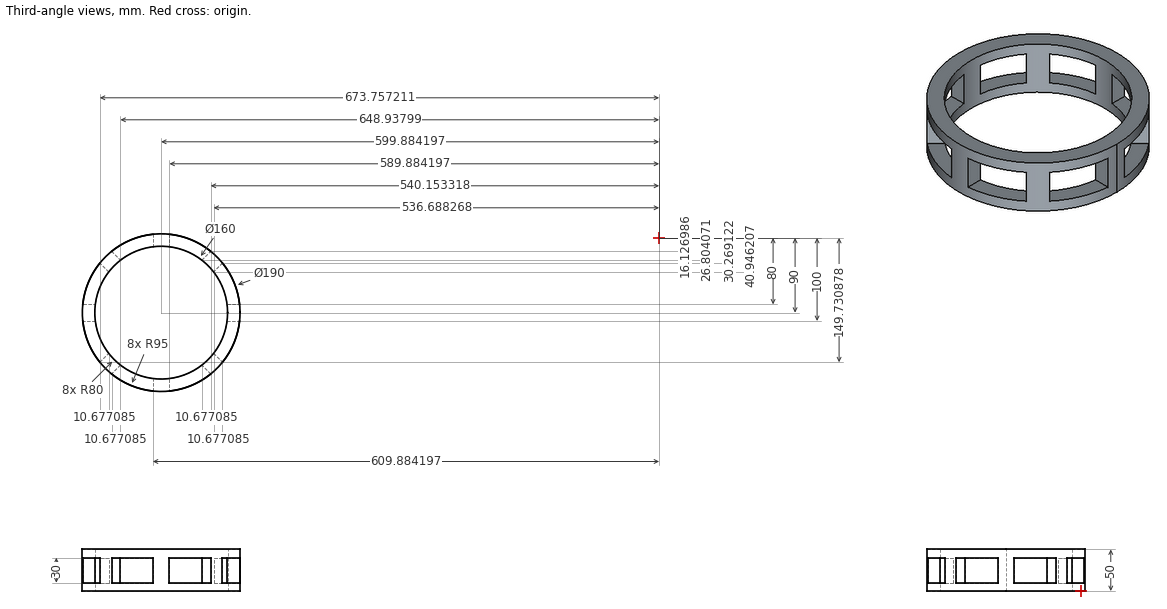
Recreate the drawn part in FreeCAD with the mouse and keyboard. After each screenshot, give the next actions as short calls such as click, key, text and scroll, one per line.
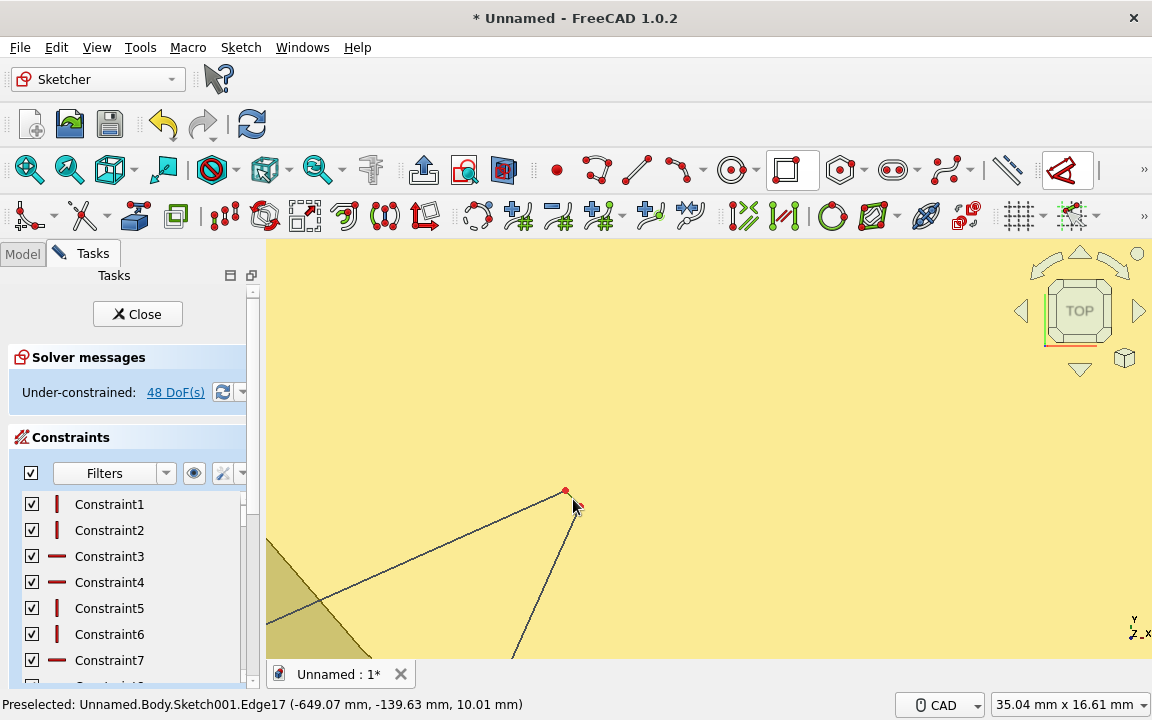
scroll(579, 512, down, 15)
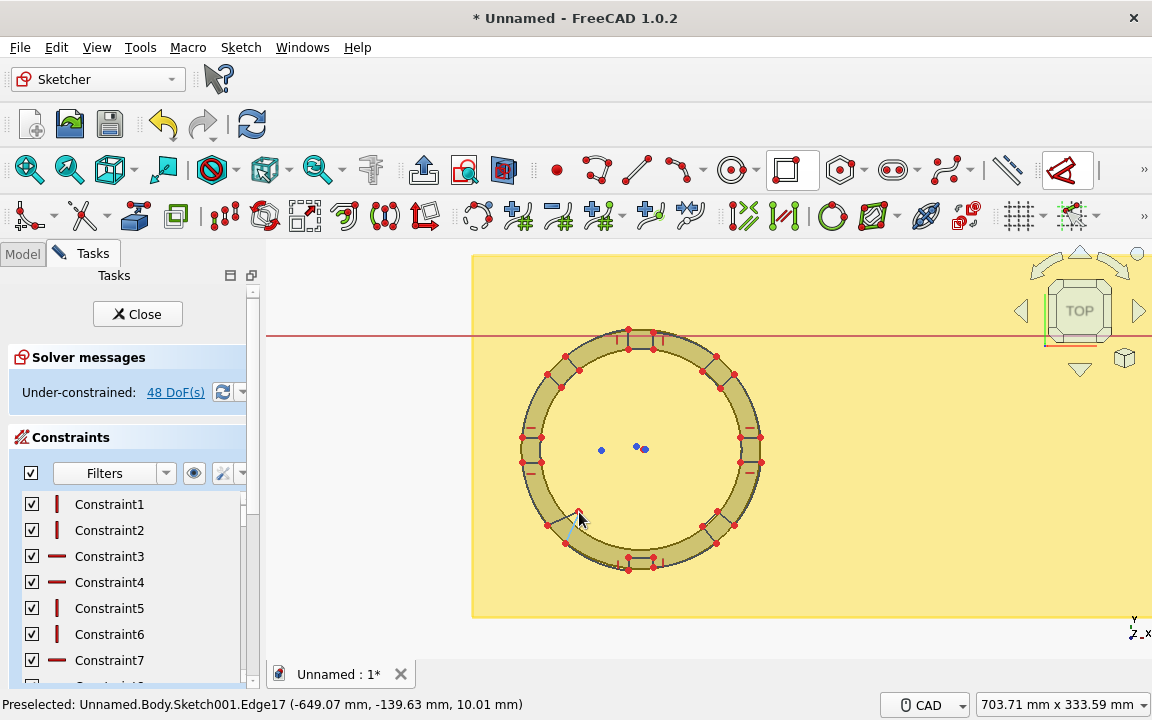
click(536, 392)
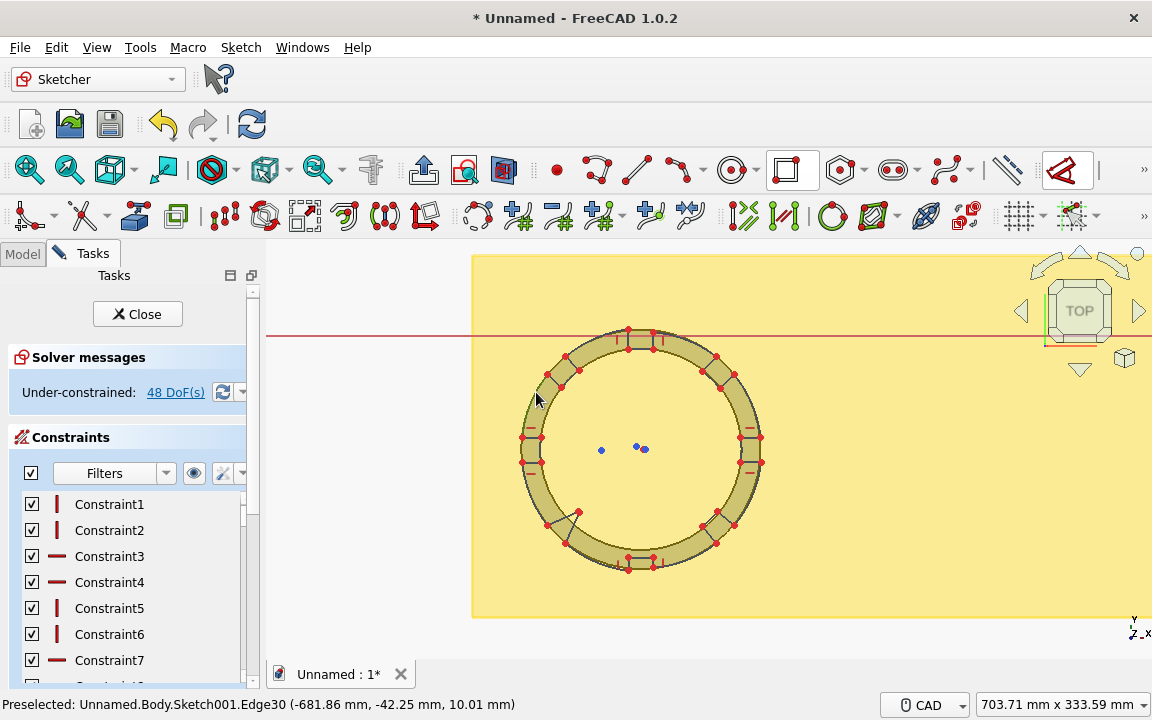
key(c)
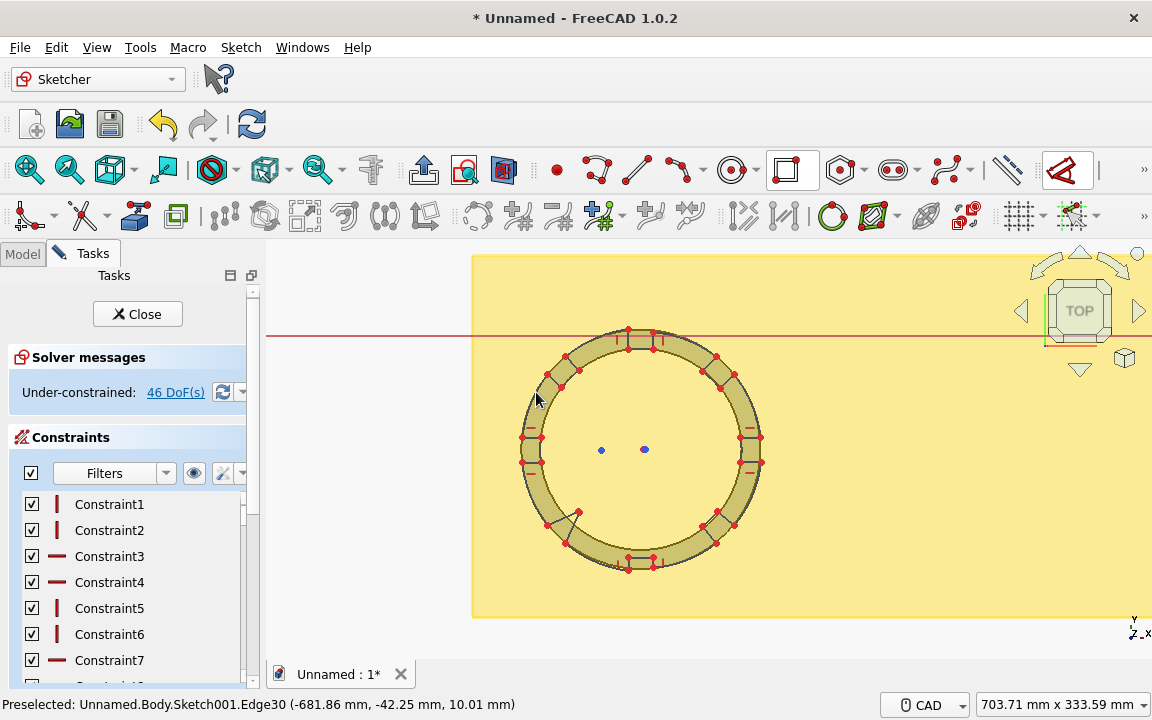
scroll(579, 512, up, 15)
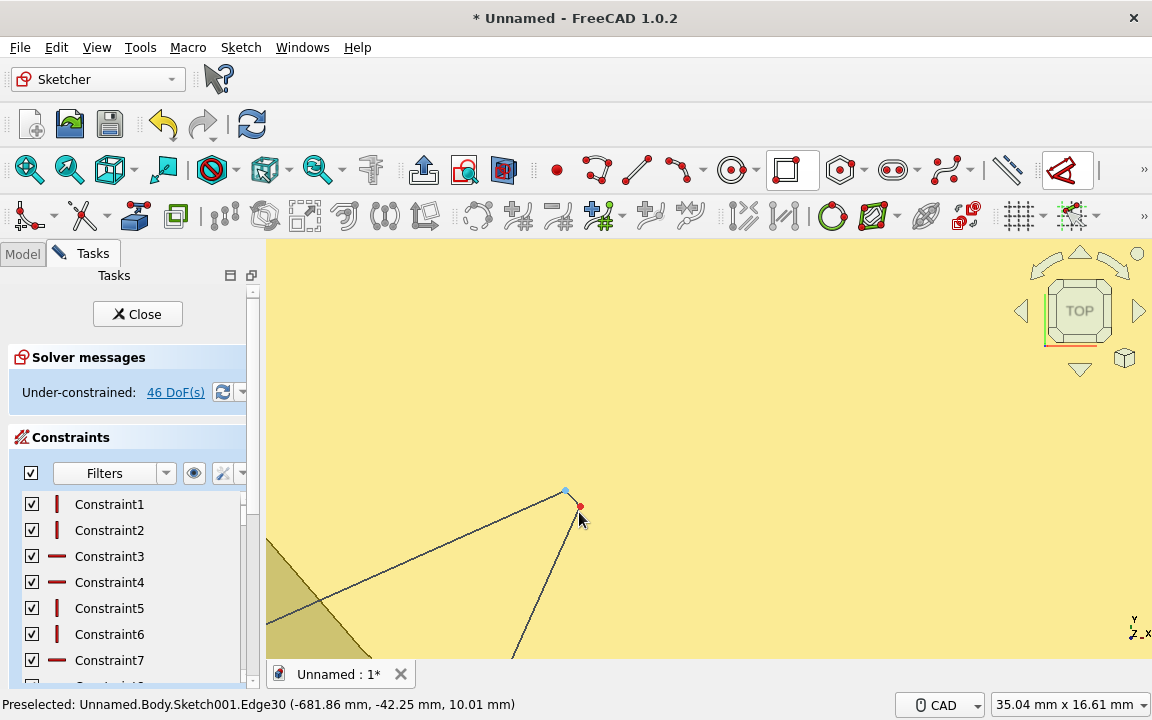
click(573, 499)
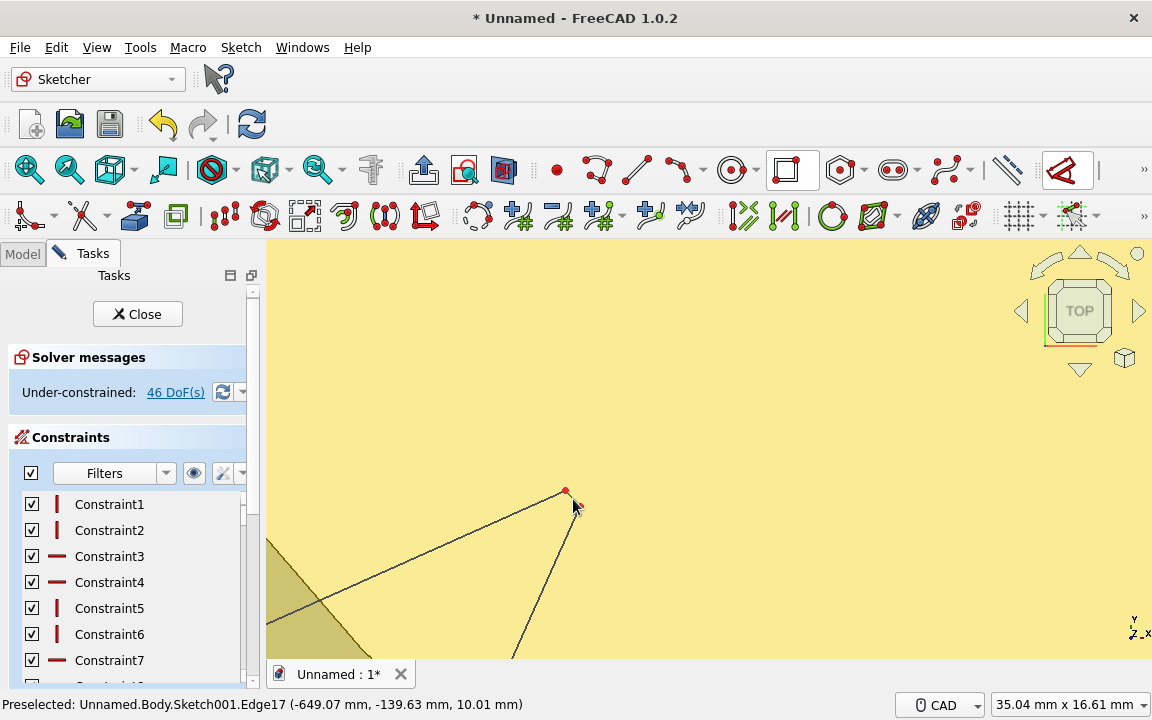
scroll(579, 512, down, 15)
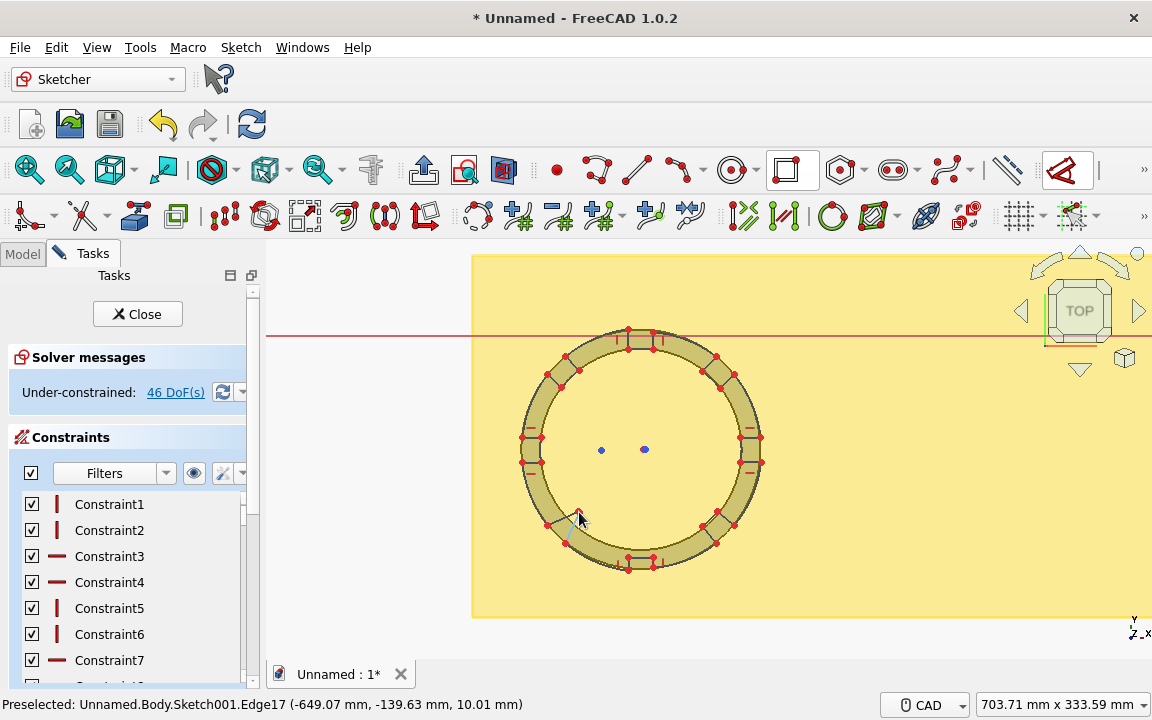
scroll(540, 445, up, 4)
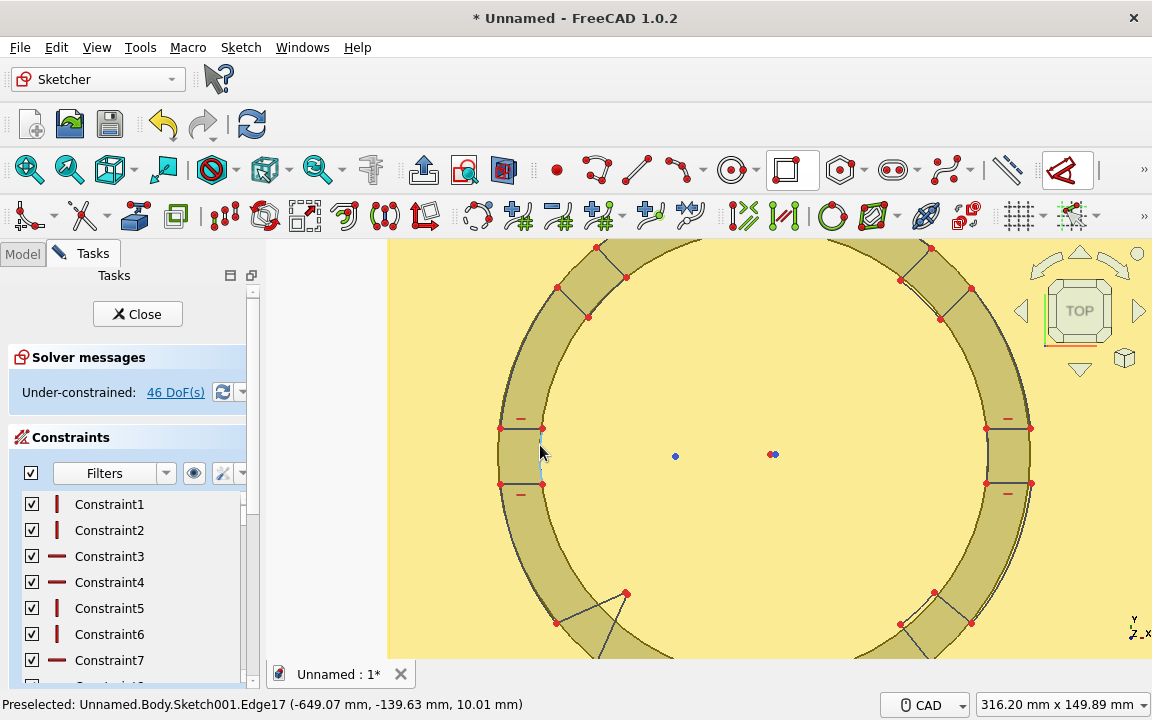
click(540, 445)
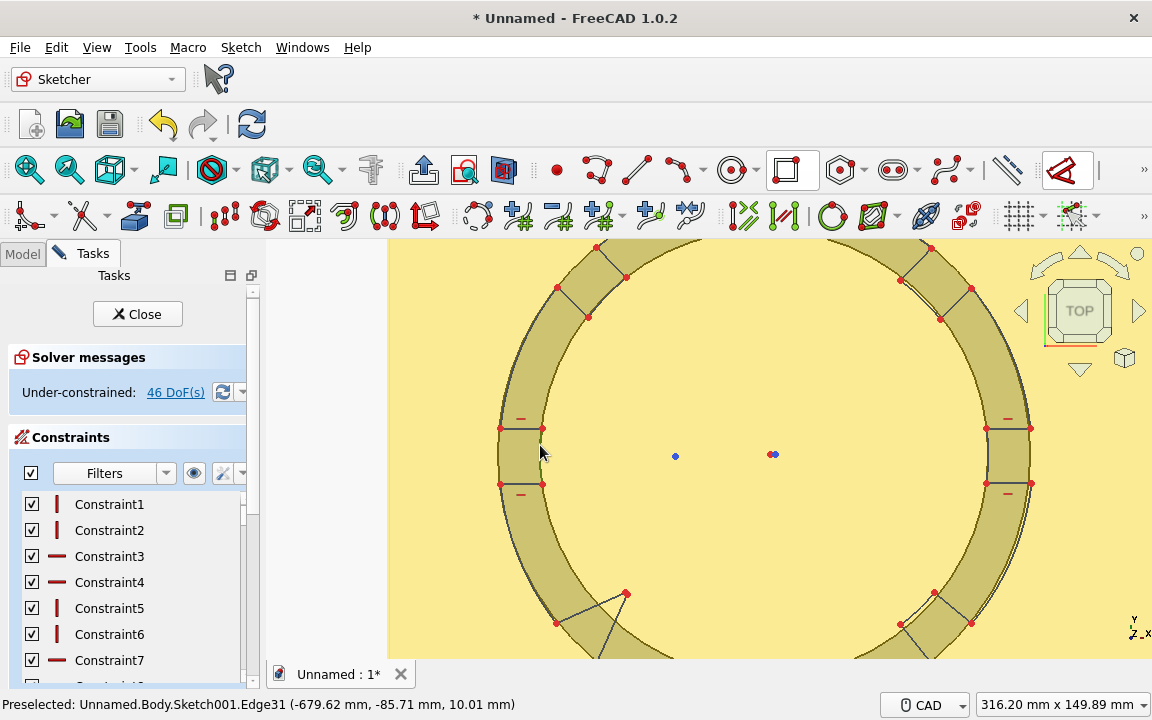
key(c)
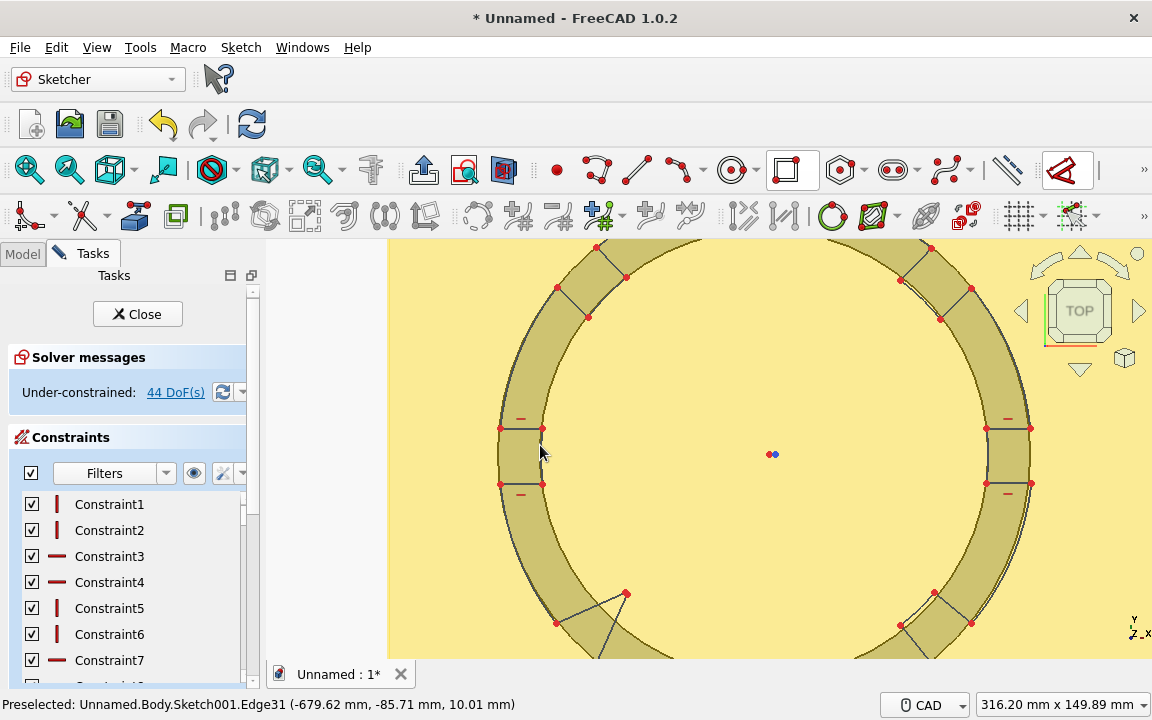
scroll(626, 593, up, 11)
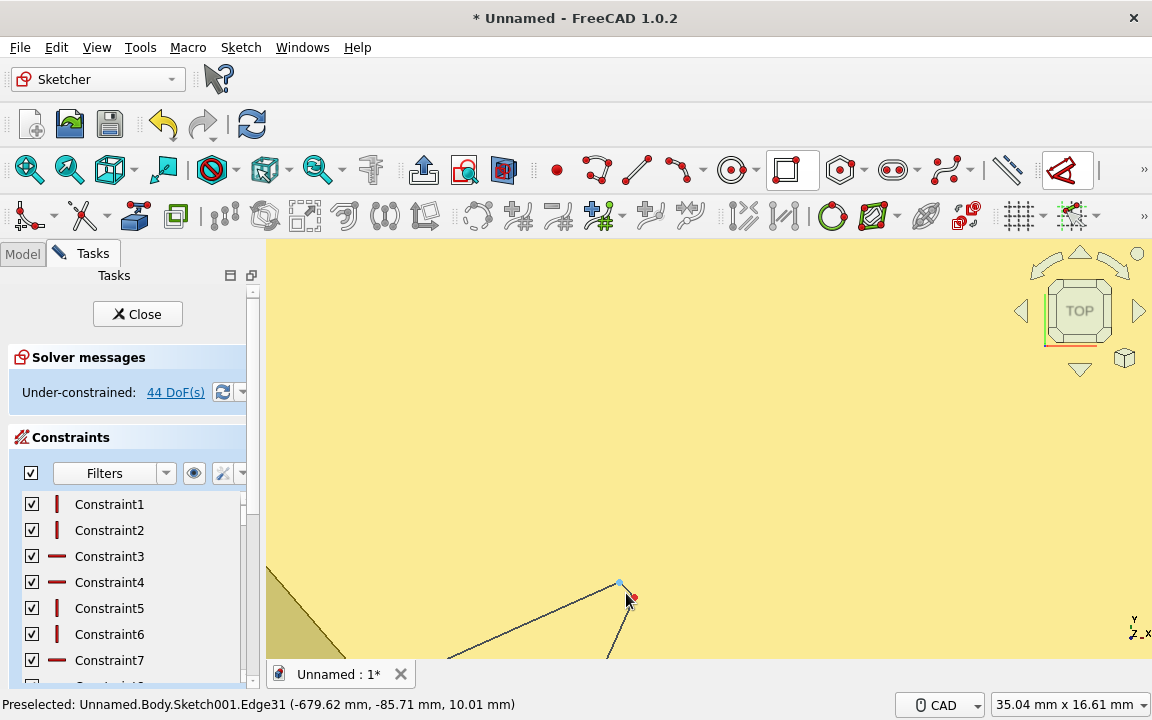
click(627, 590)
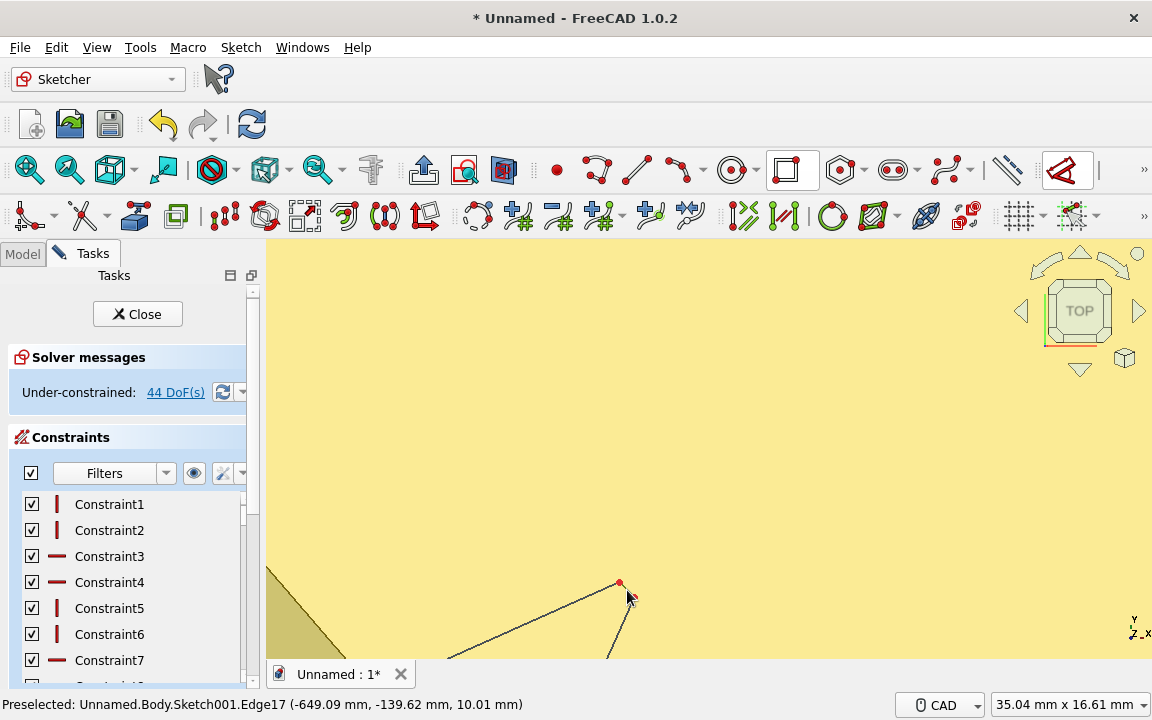
scroll(576, 508, down, 15)